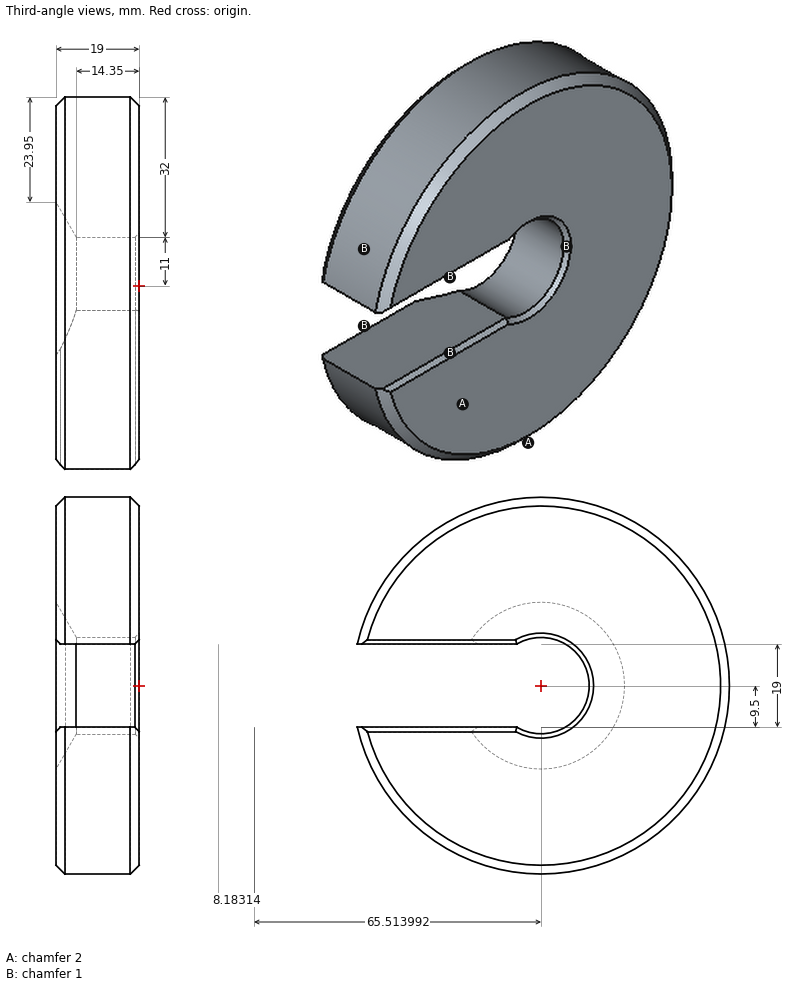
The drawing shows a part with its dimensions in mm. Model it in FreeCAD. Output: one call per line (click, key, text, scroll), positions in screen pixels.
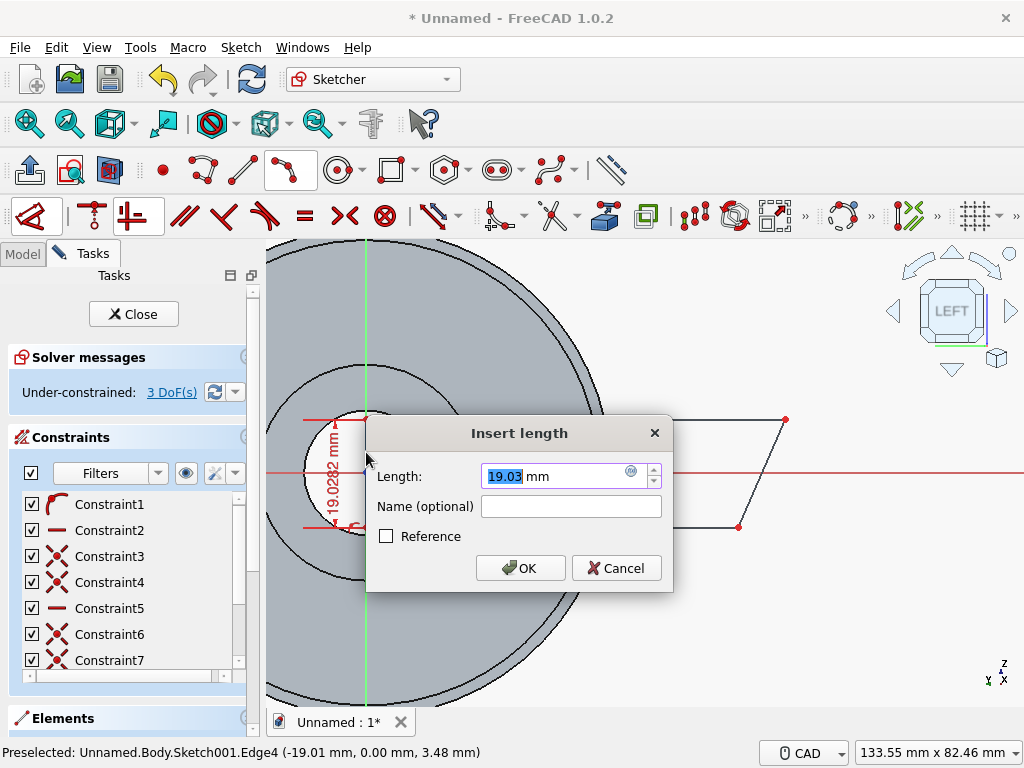
text(19)
key(Return)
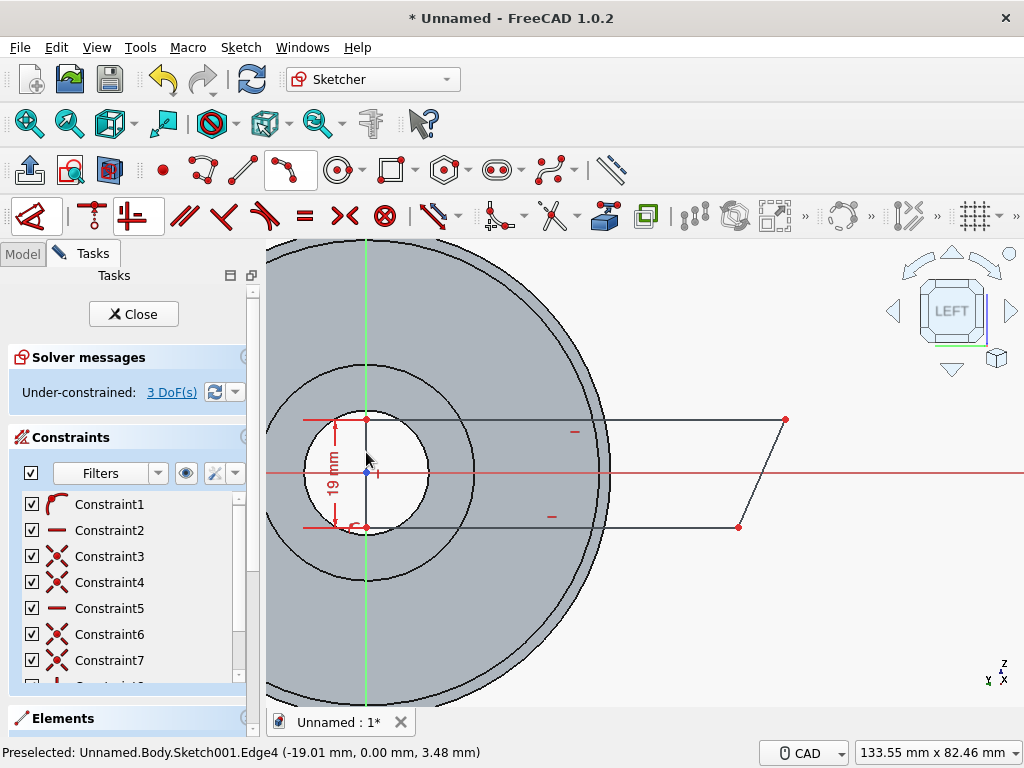
click(366, 528)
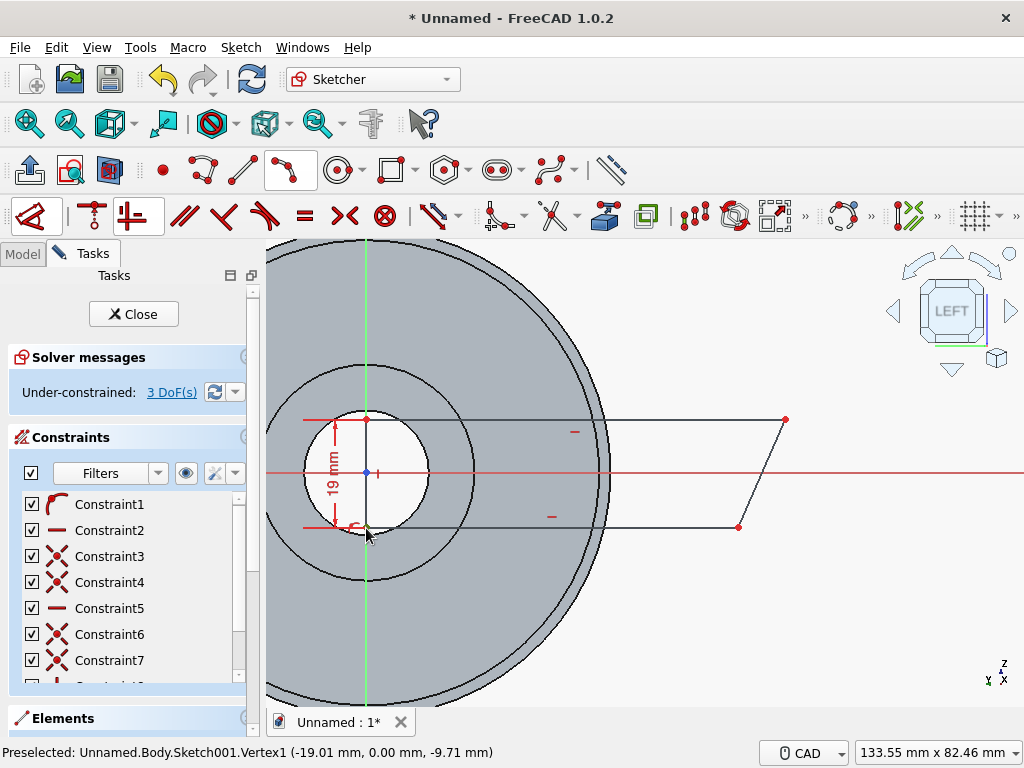
click(56, 216)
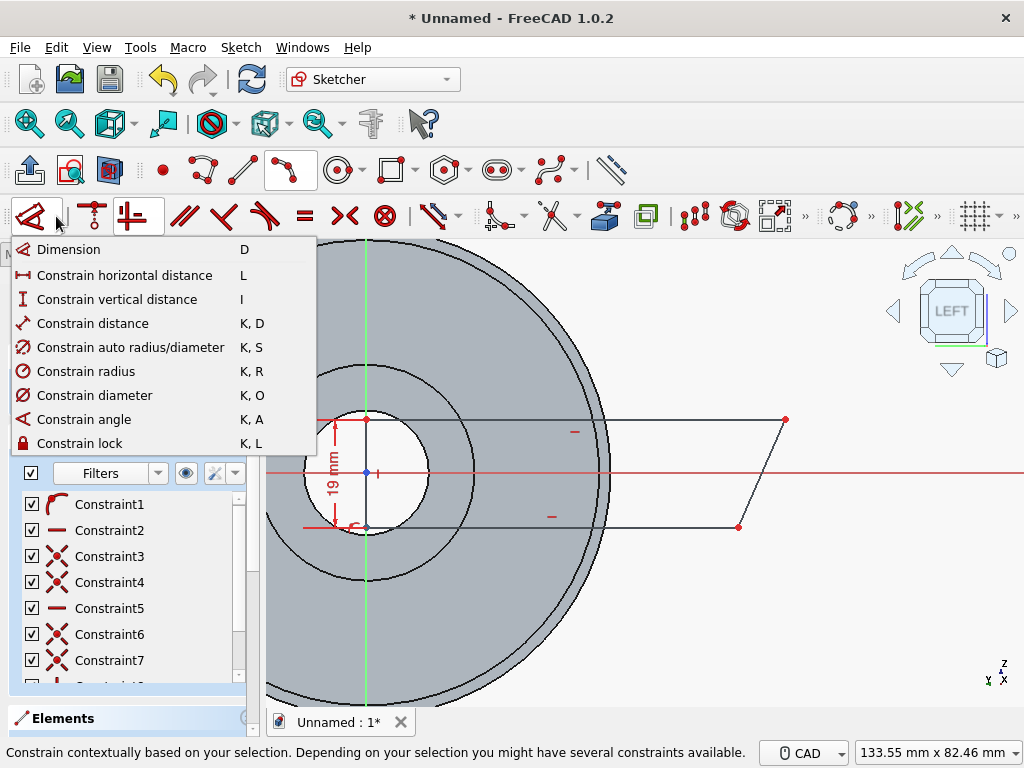
click(164, 299)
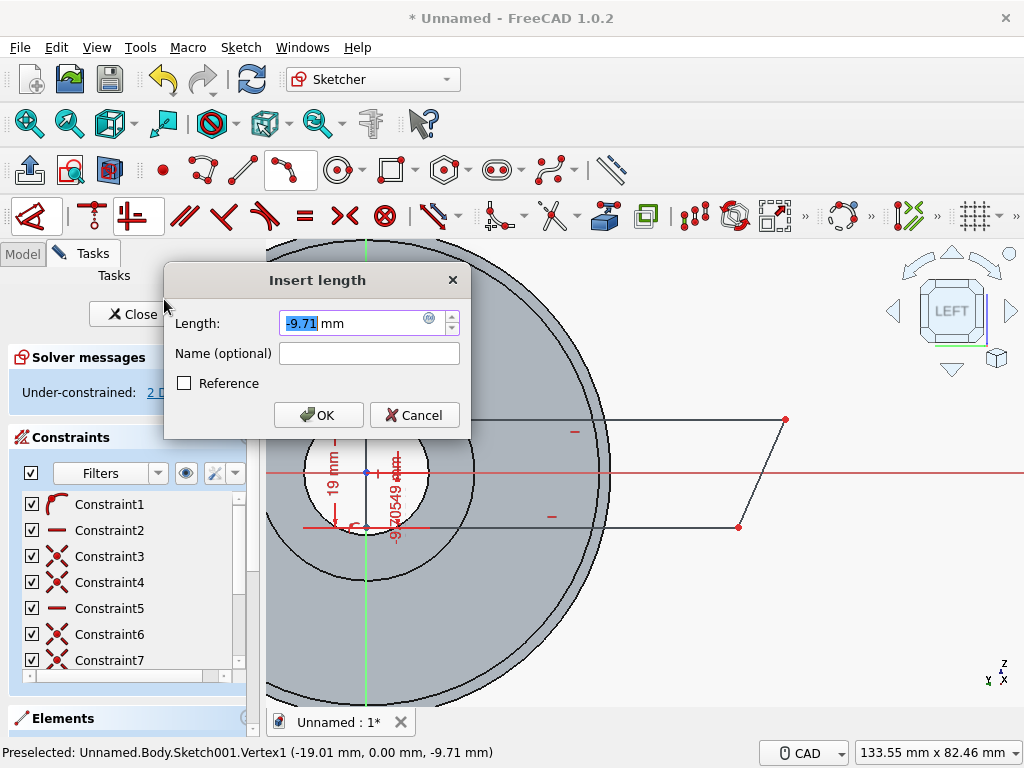
text(-9.5)
key(Return)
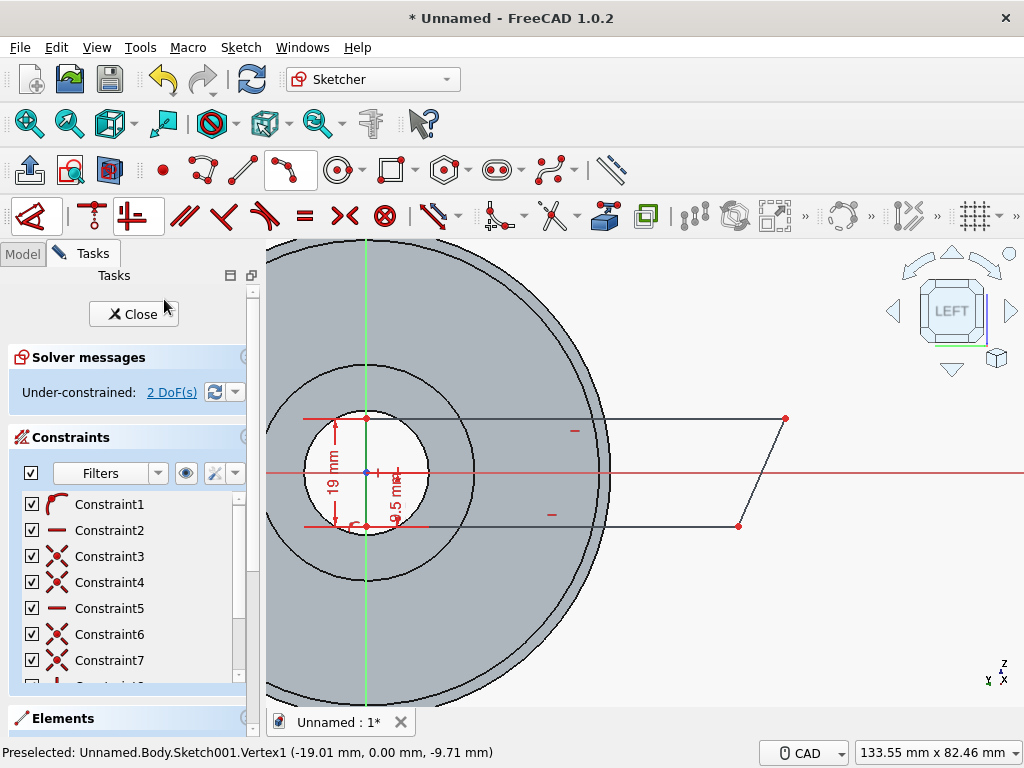
click(752, 494)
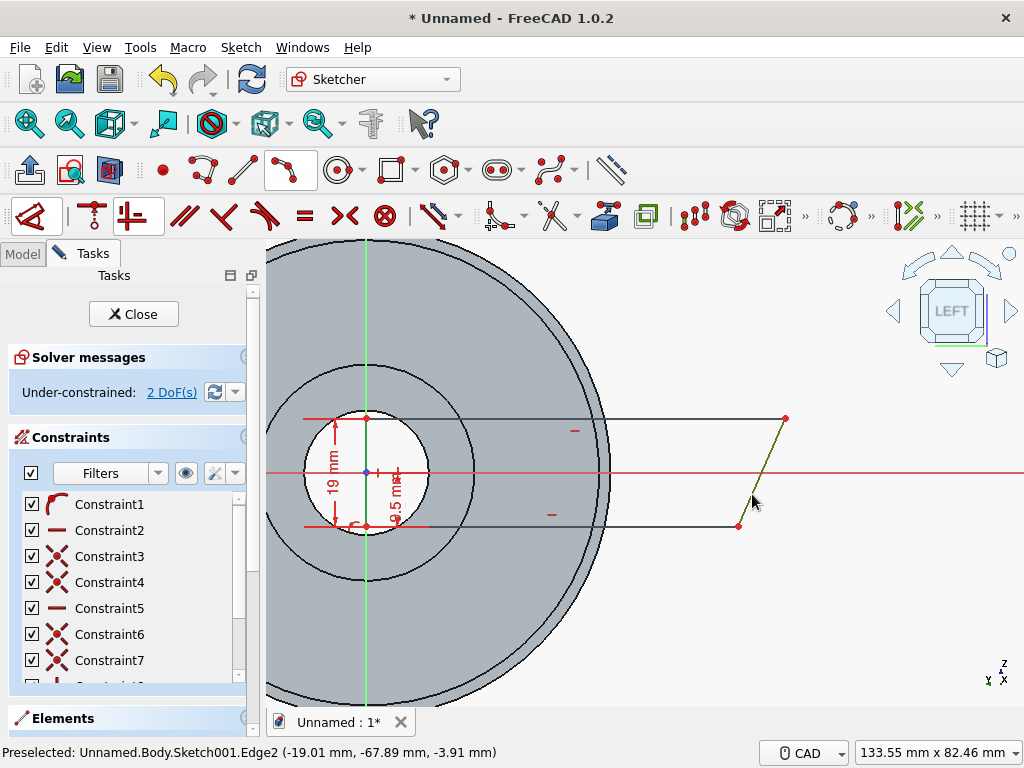
key(l)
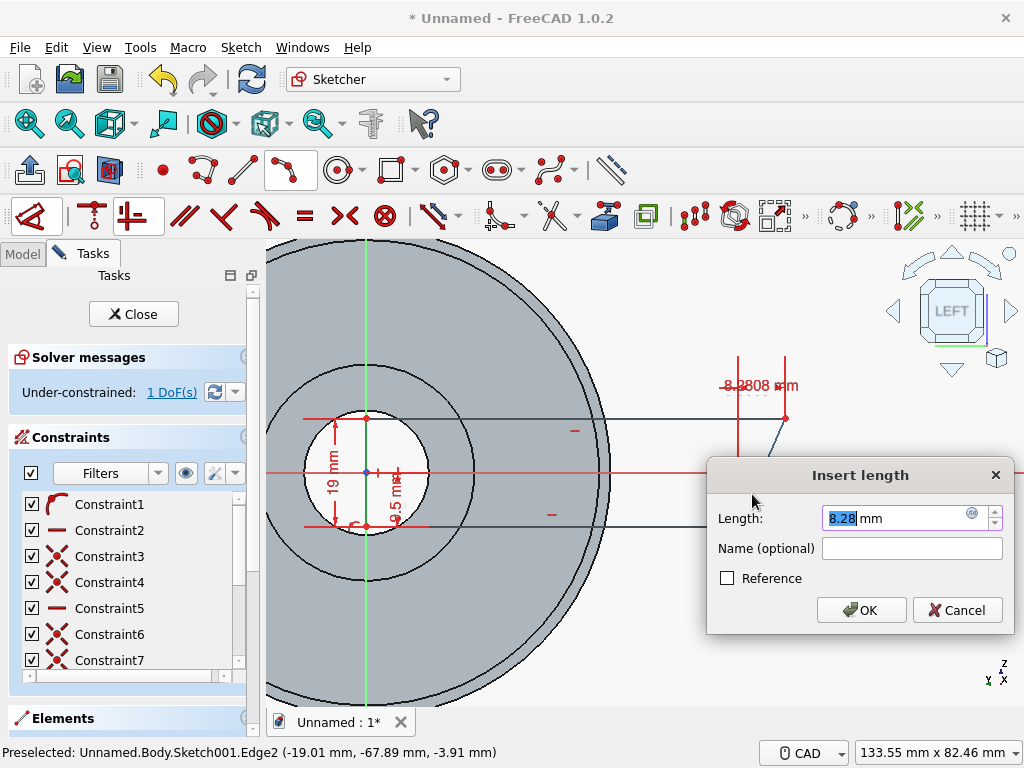
text(8.18314)
key(Return)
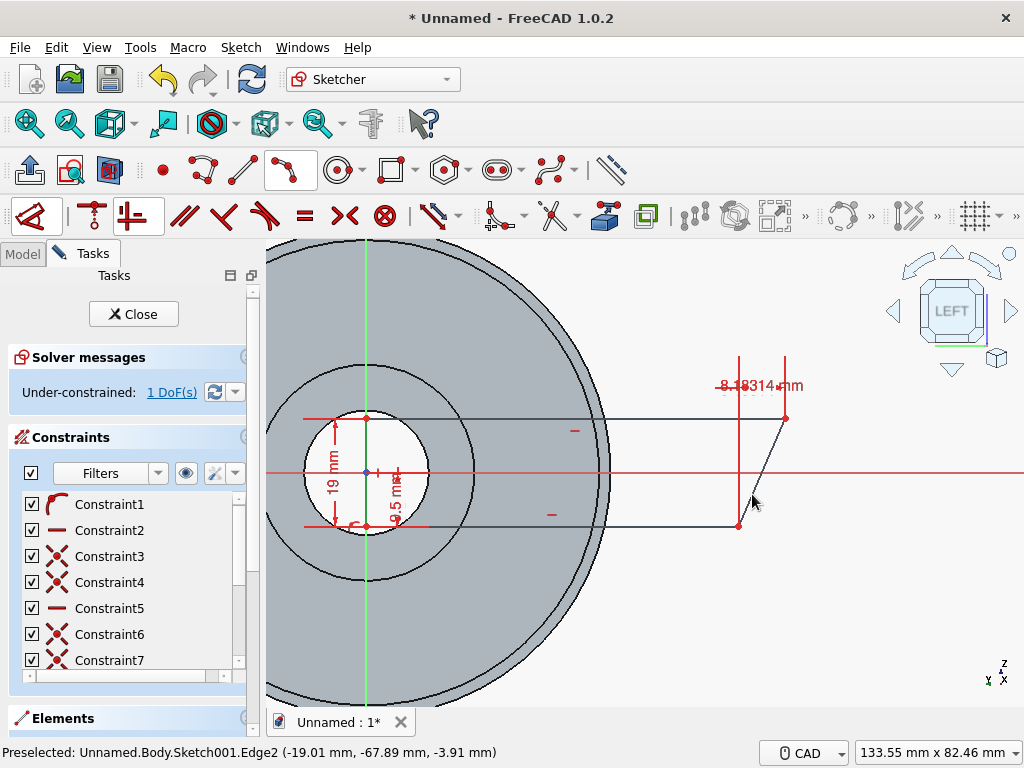
click(478, 527)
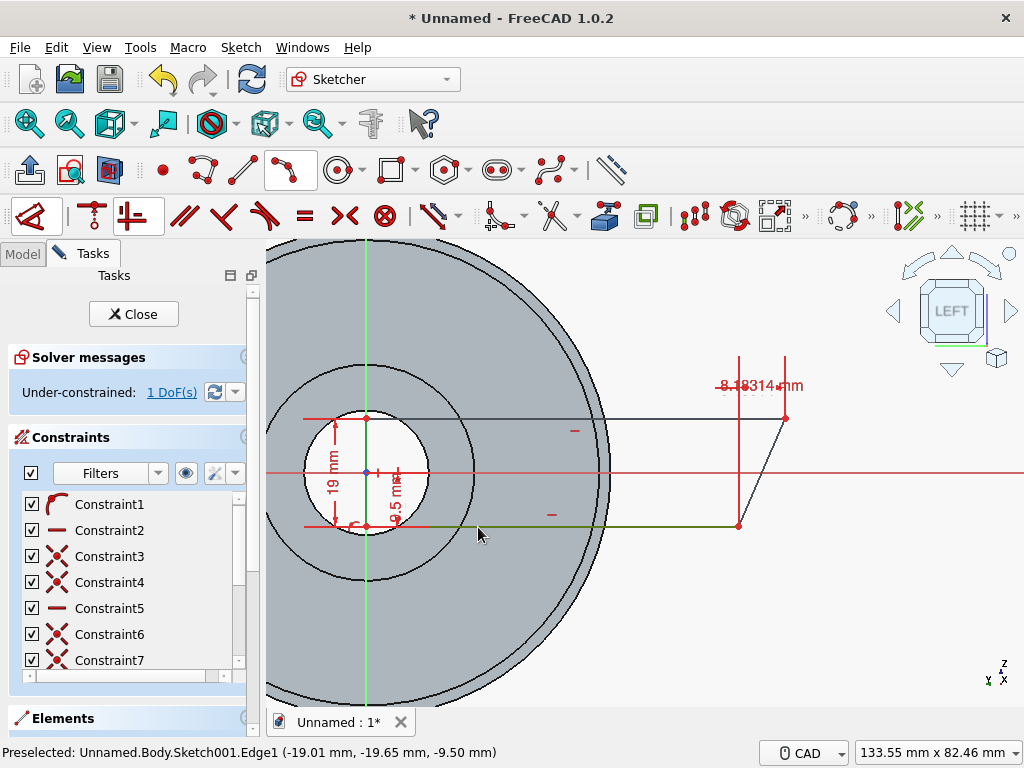
key(l)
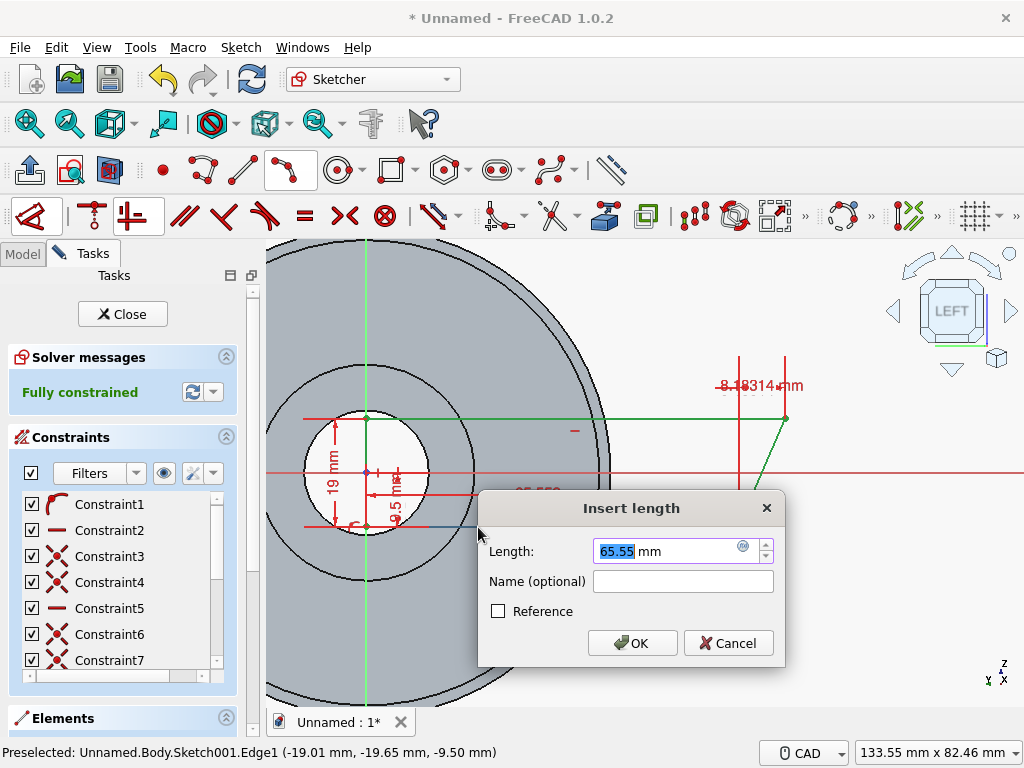
text(65.513992)
key(Return)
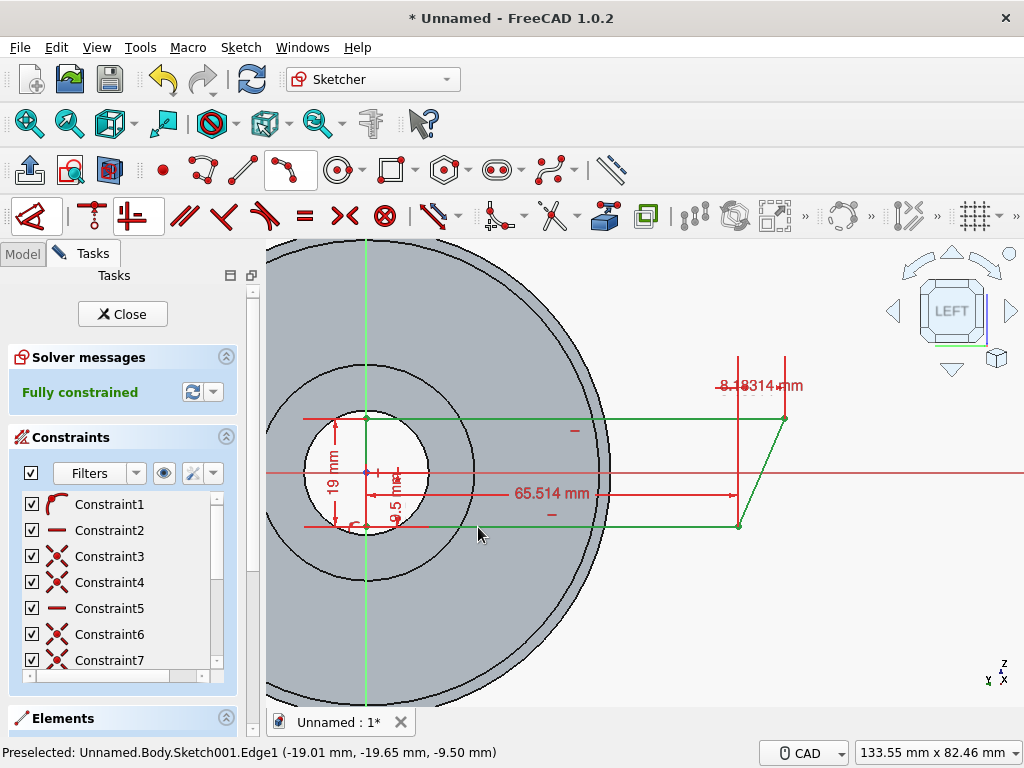
click(123, 314)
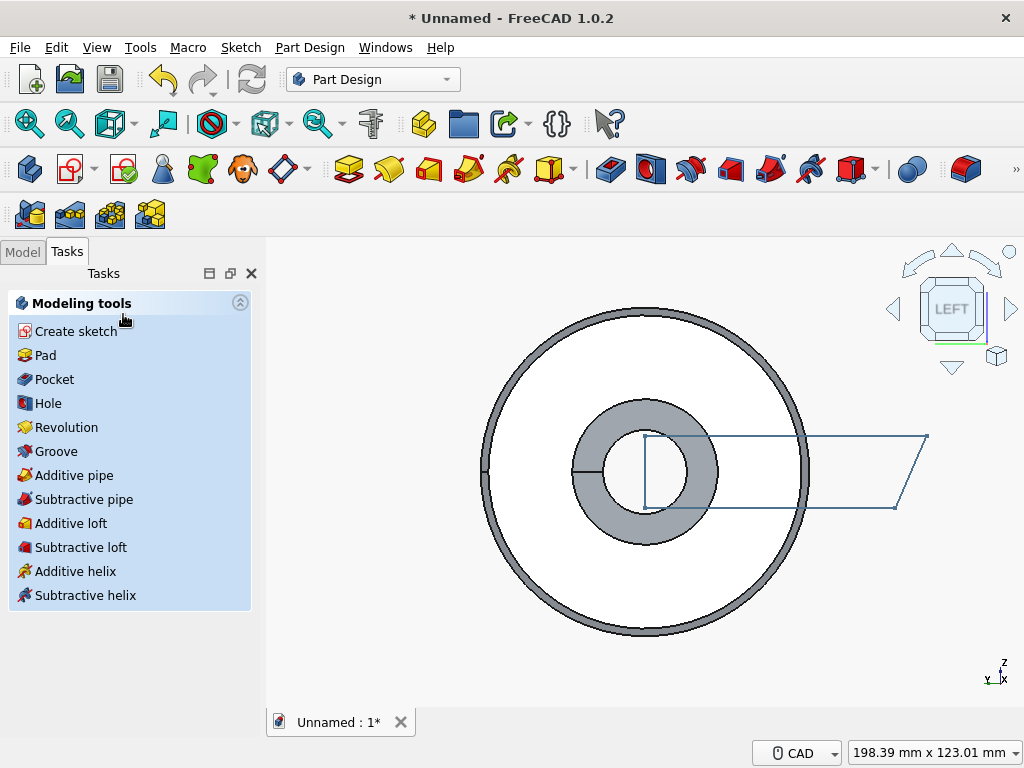
click(612, 170)